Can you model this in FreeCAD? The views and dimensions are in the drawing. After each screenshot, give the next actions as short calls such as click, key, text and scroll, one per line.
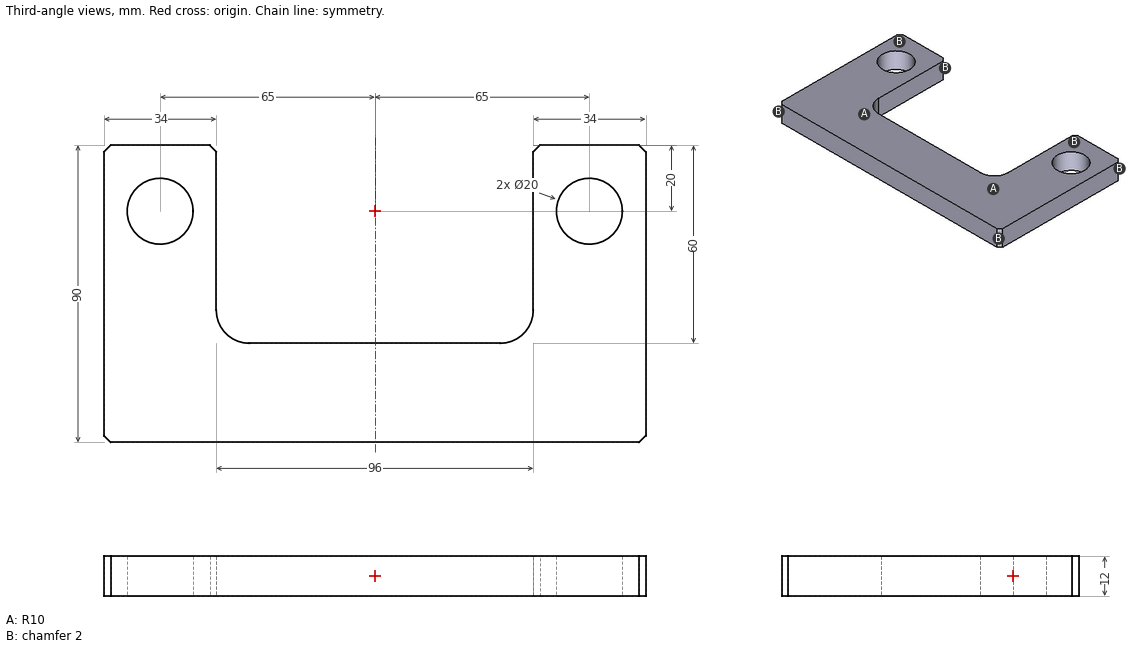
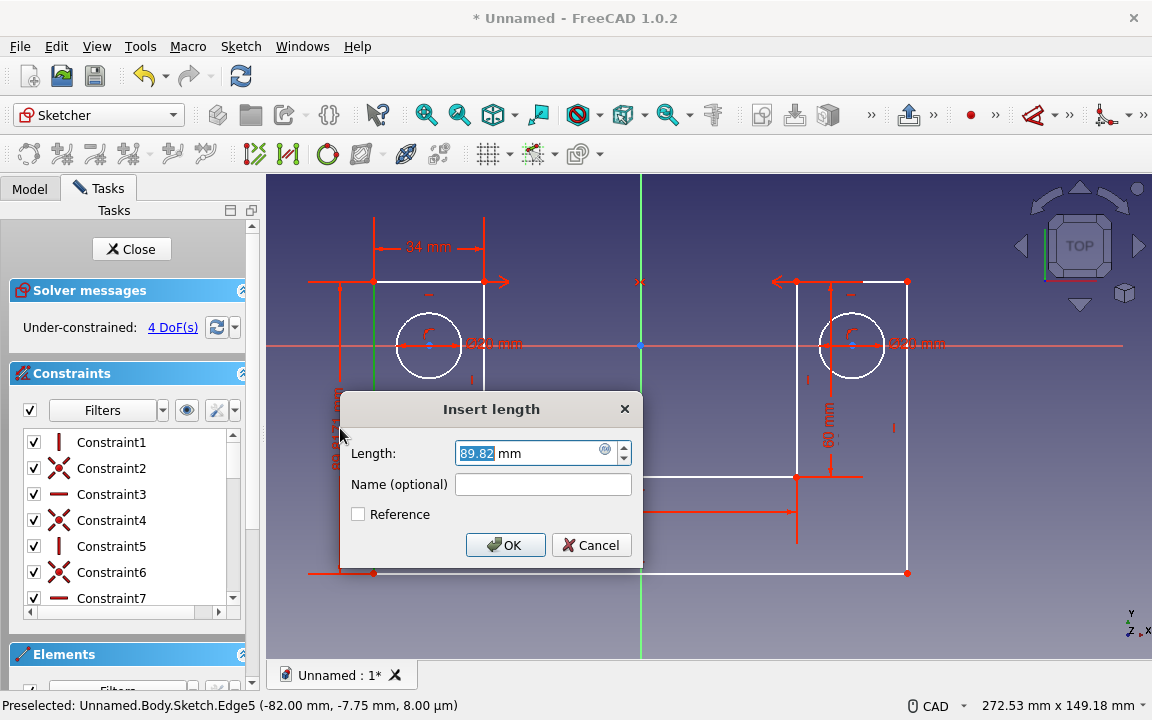
text(90)
key(Return)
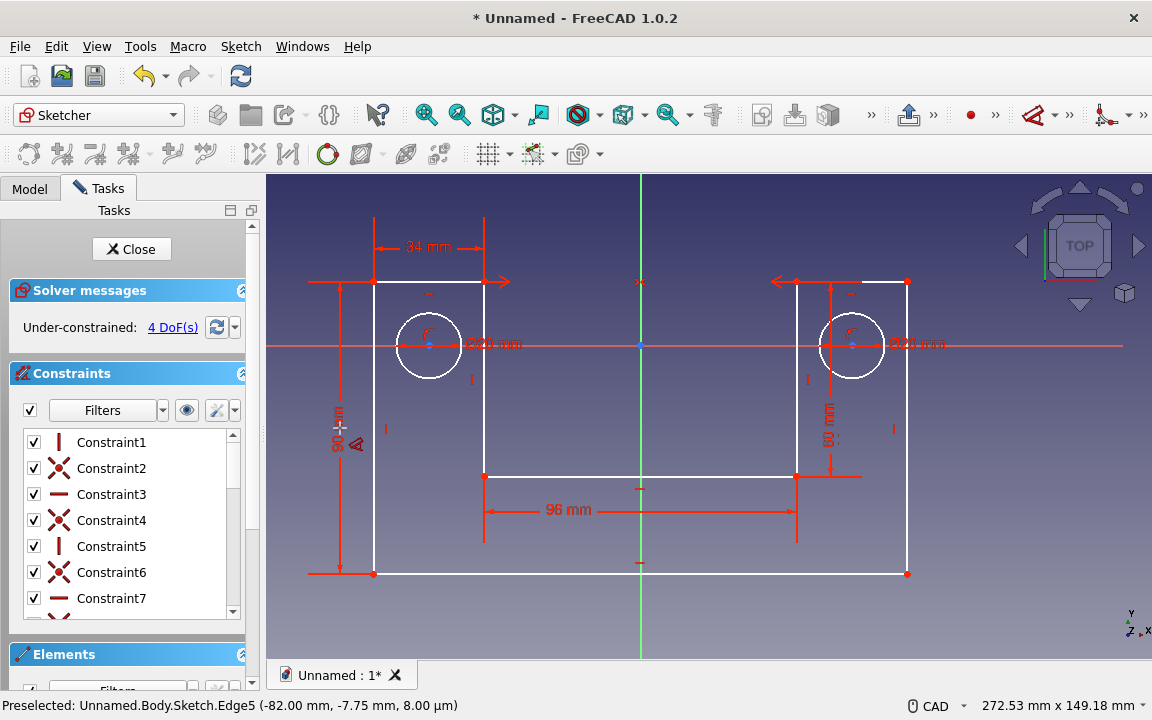
click(874, 282)
click(852, 248)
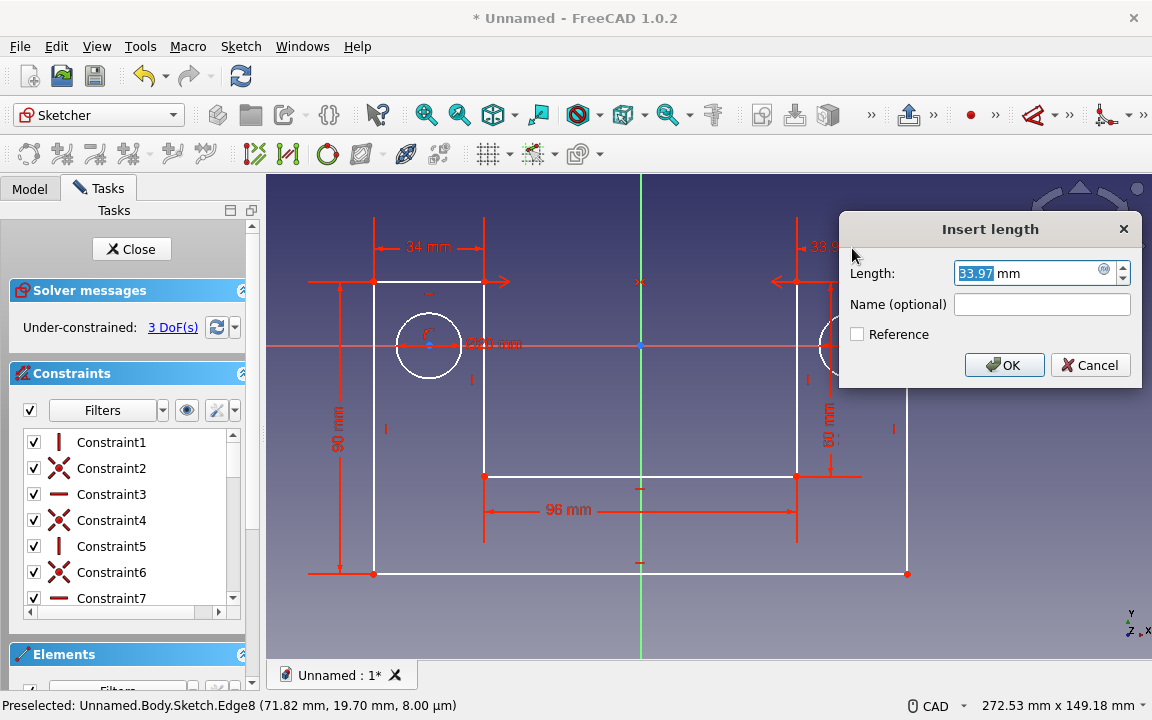
text(34)
key(Return)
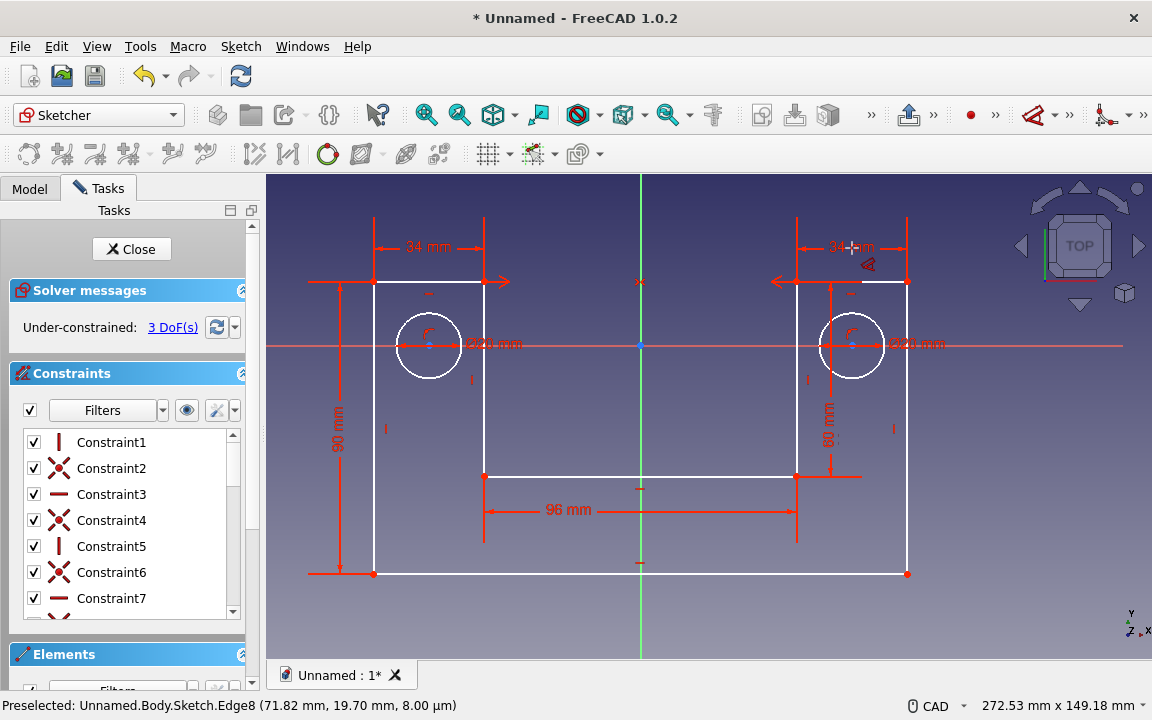
click(852, 346)
click(746, 312)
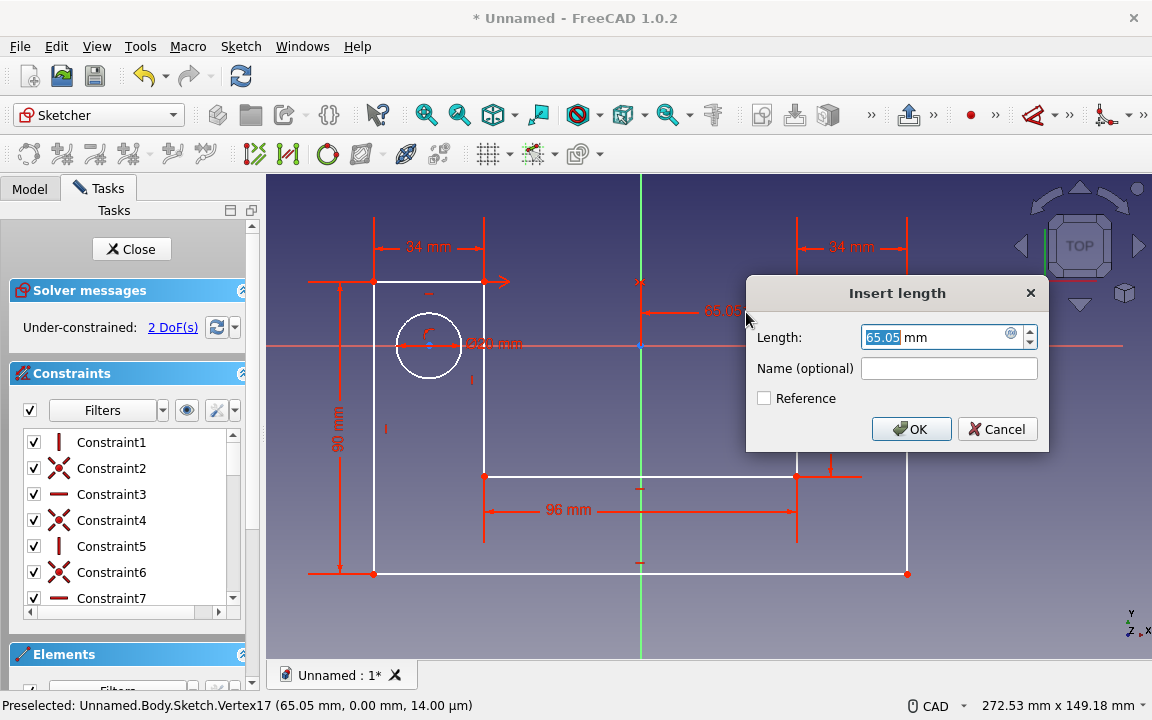
text(65)
key(Return)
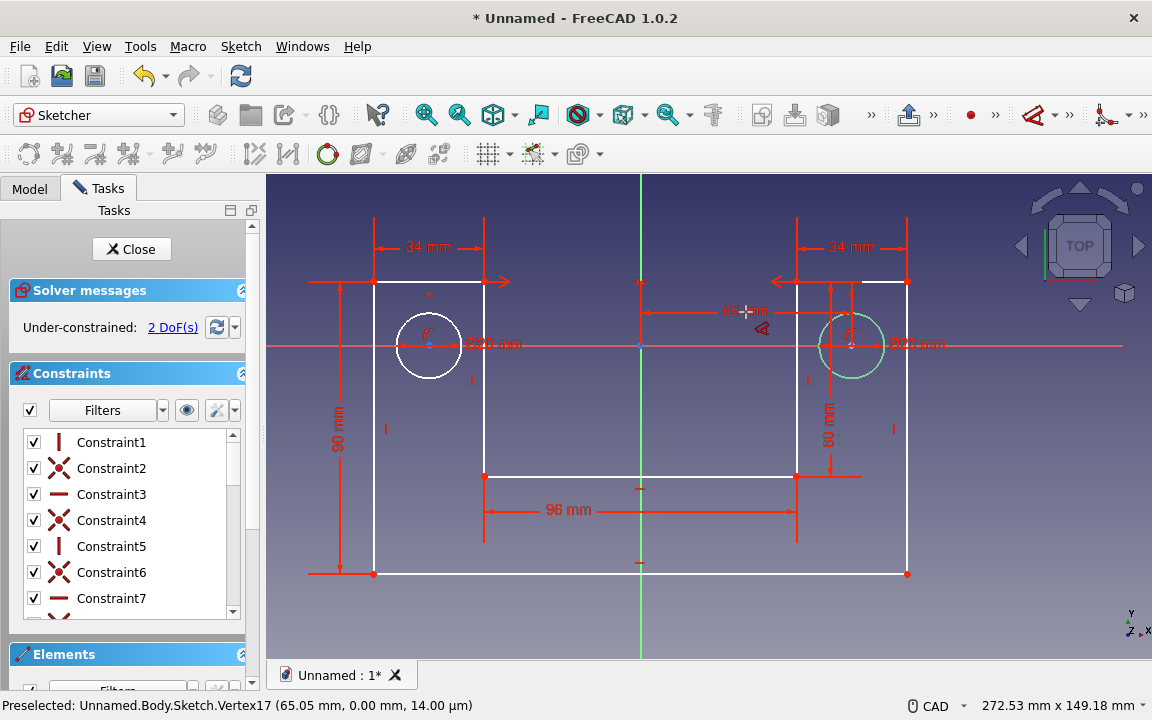
click(429, 346)
click(535, 312)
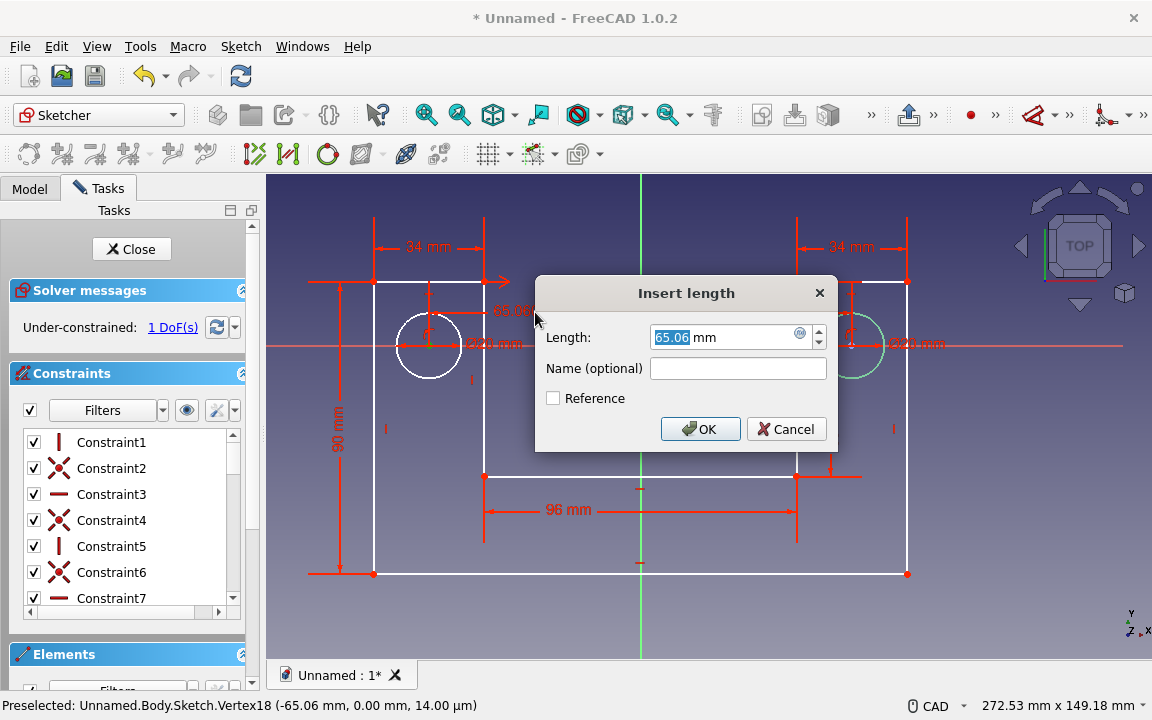
text(65)
key(Return)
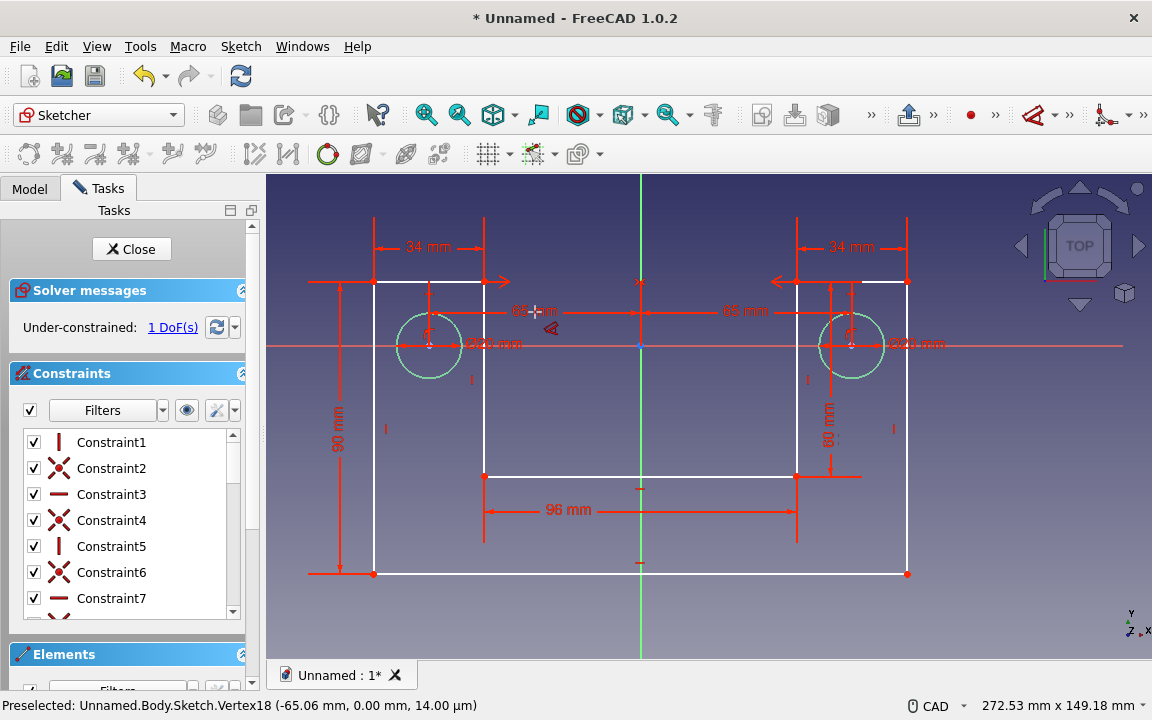
click(797, 282)
click(831, 299)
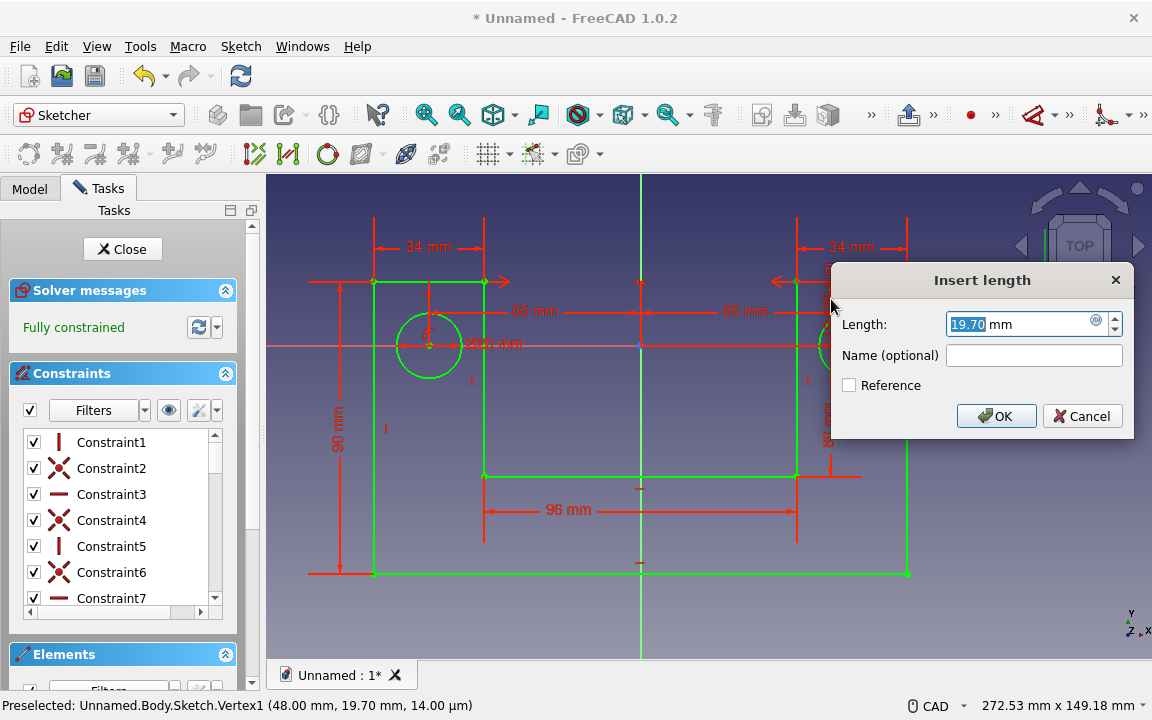
text(20)
key(Return)
key(Escape)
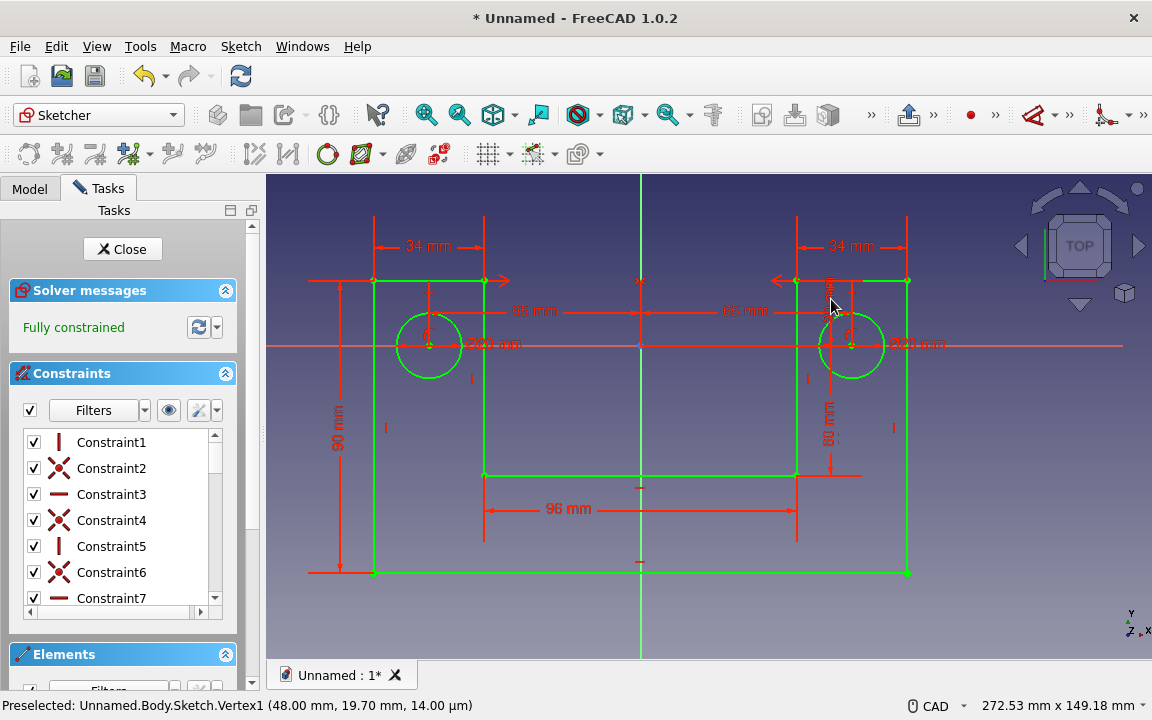
click(123, 249)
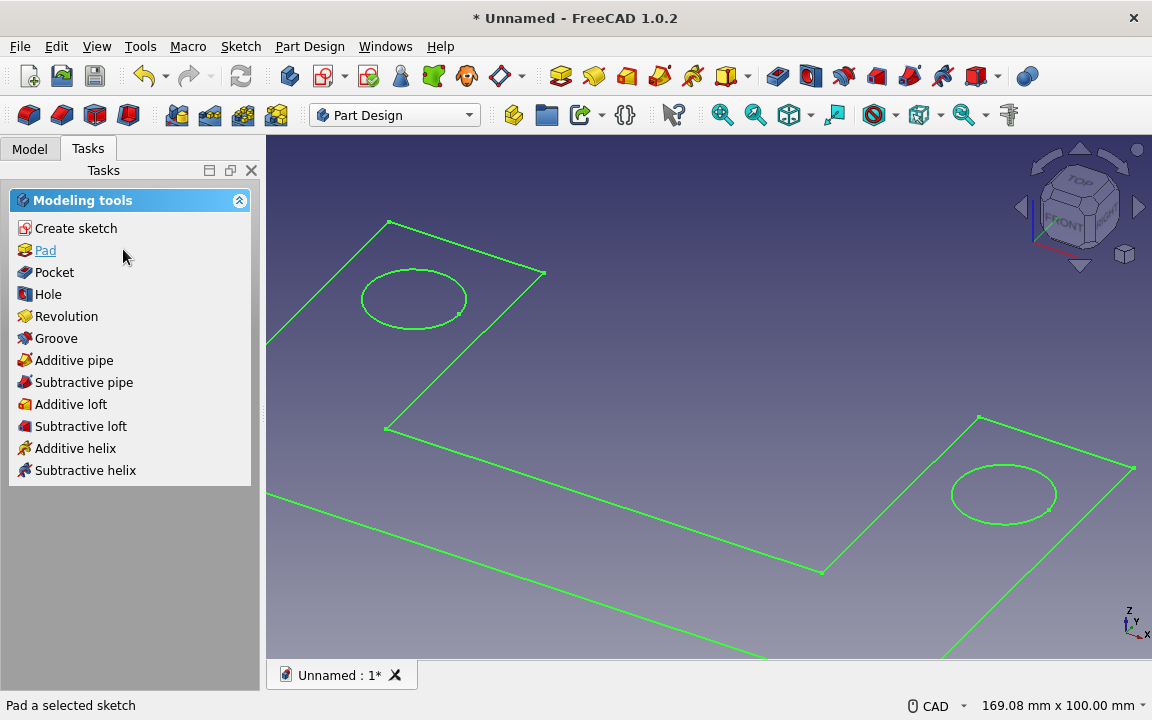
click(561, 76)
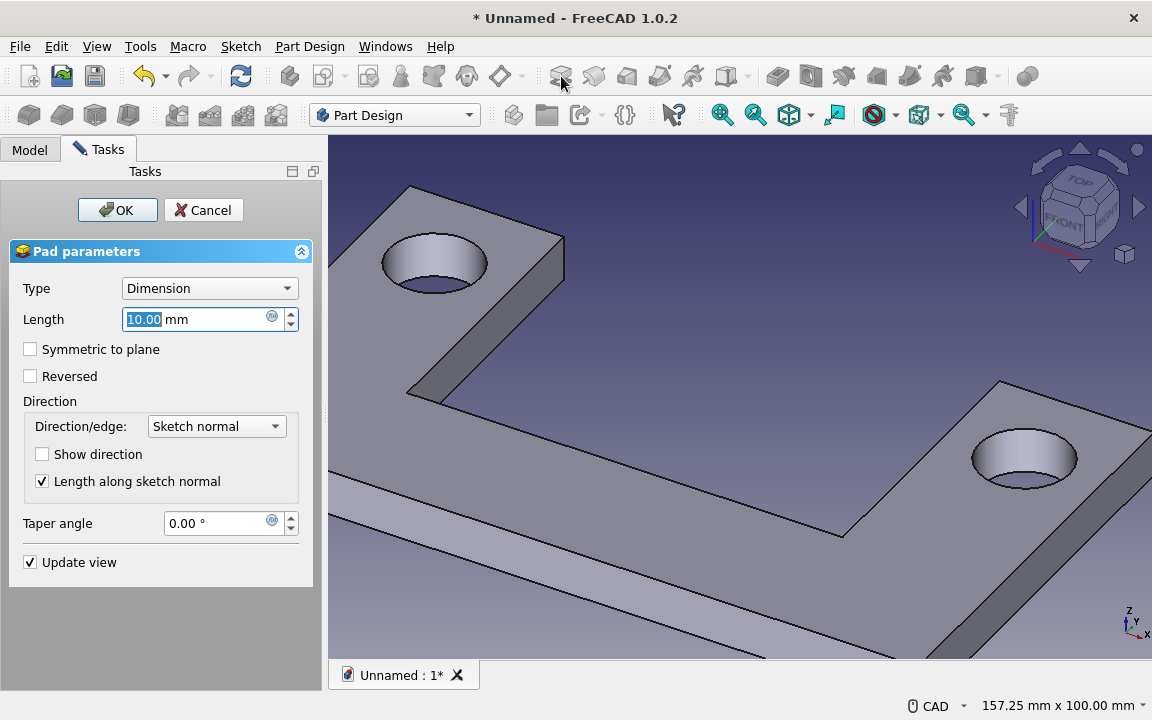
text(12)
key(Tab)